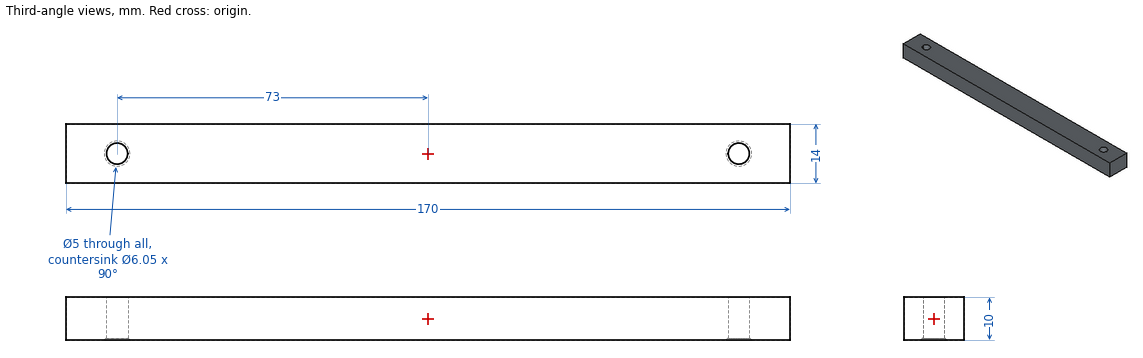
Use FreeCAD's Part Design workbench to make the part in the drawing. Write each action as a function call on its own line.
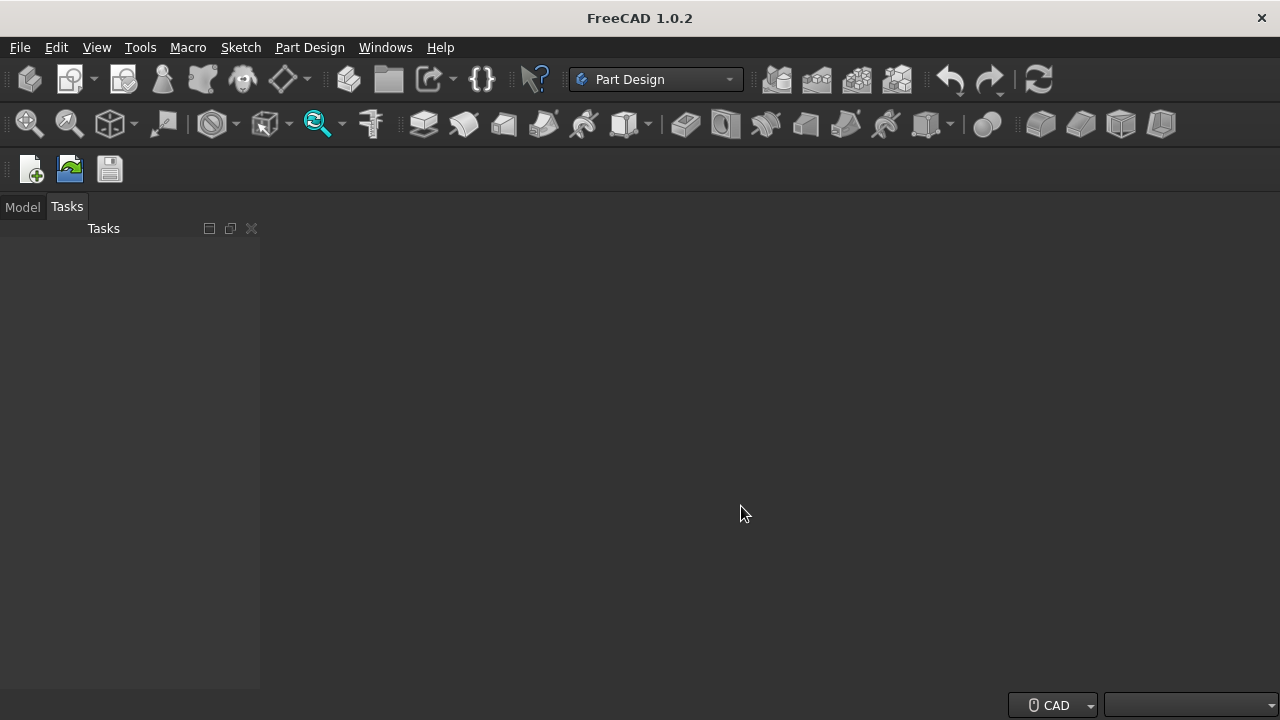
click(30, 170)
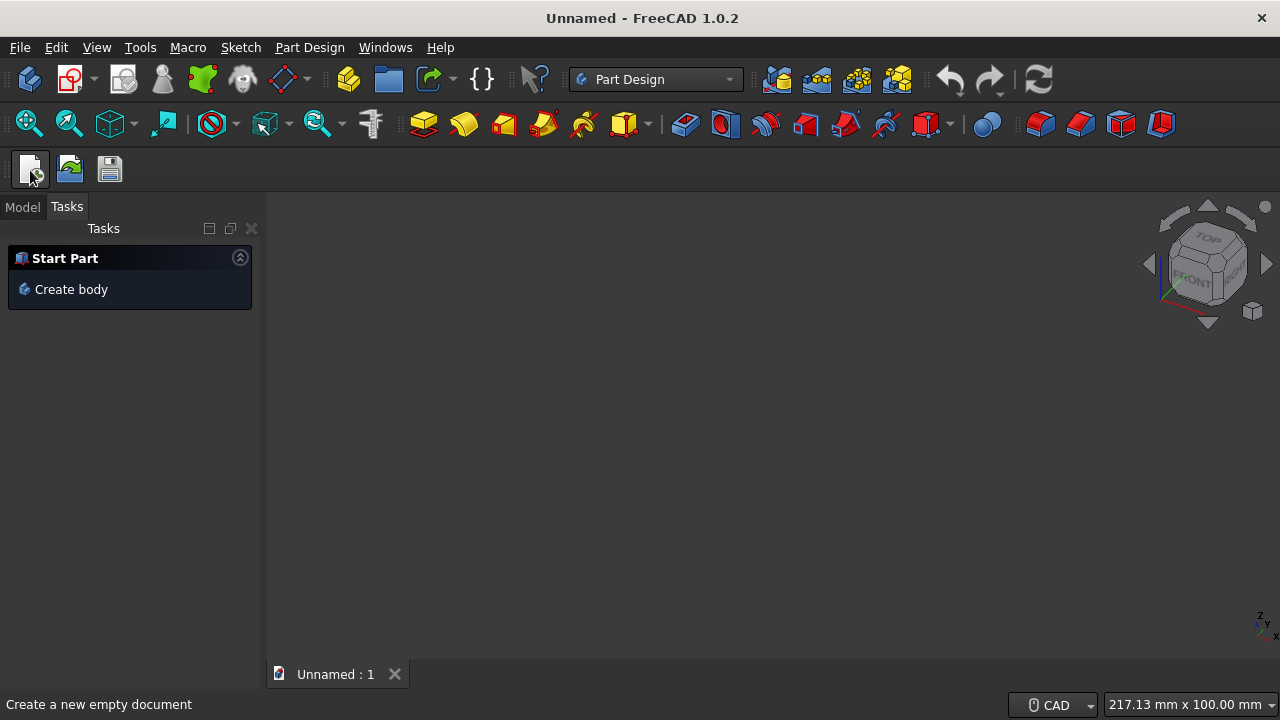
click(70, 80)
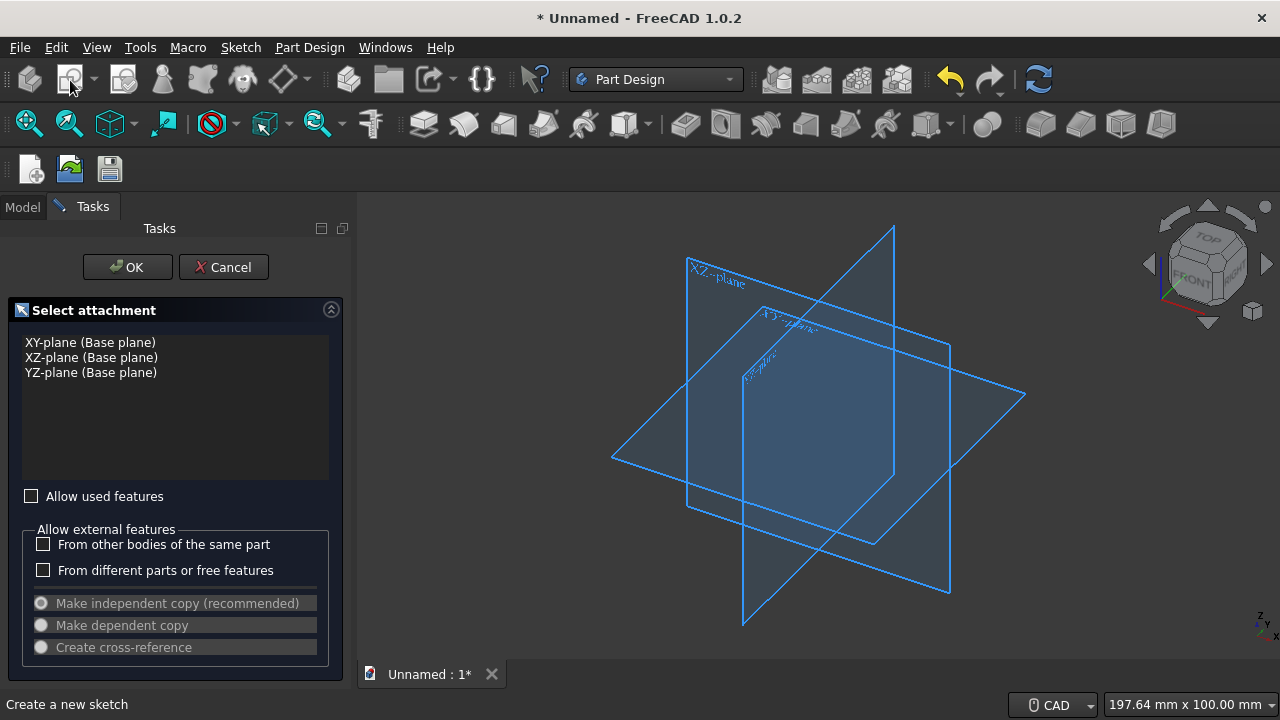
click(82, 342)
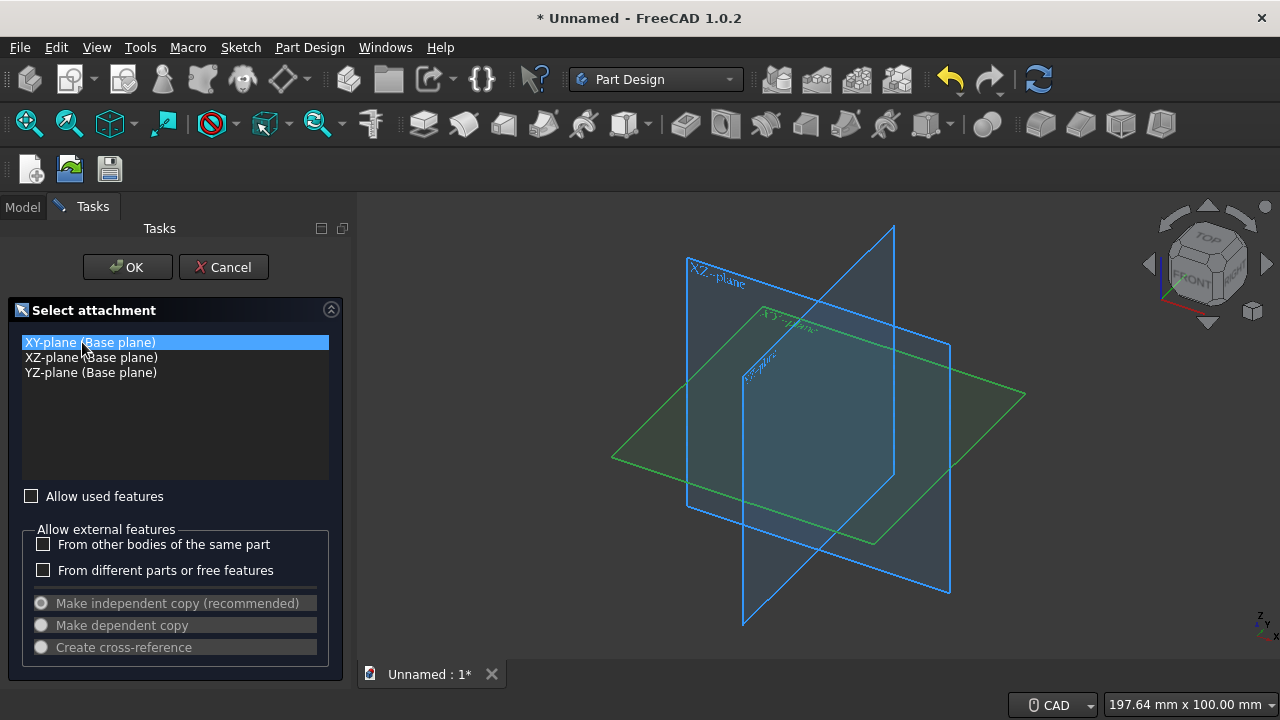
click(128, 267)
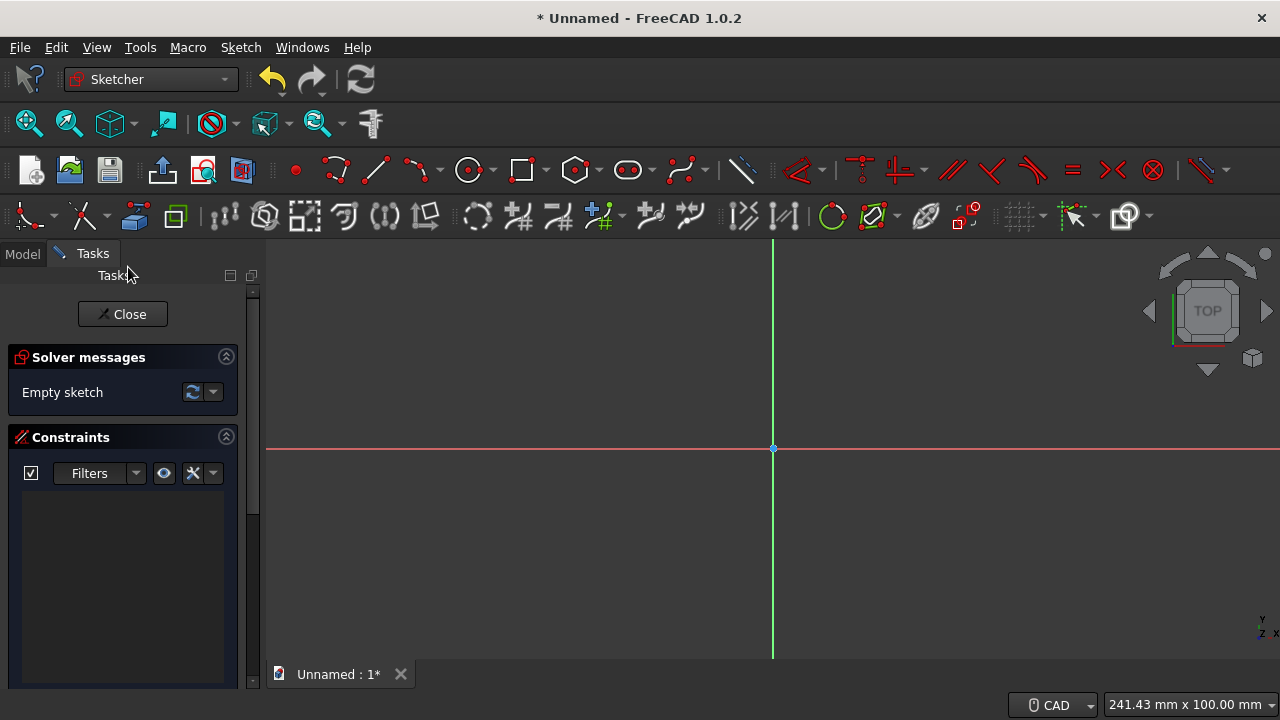
scroll(395, 449, down, 1)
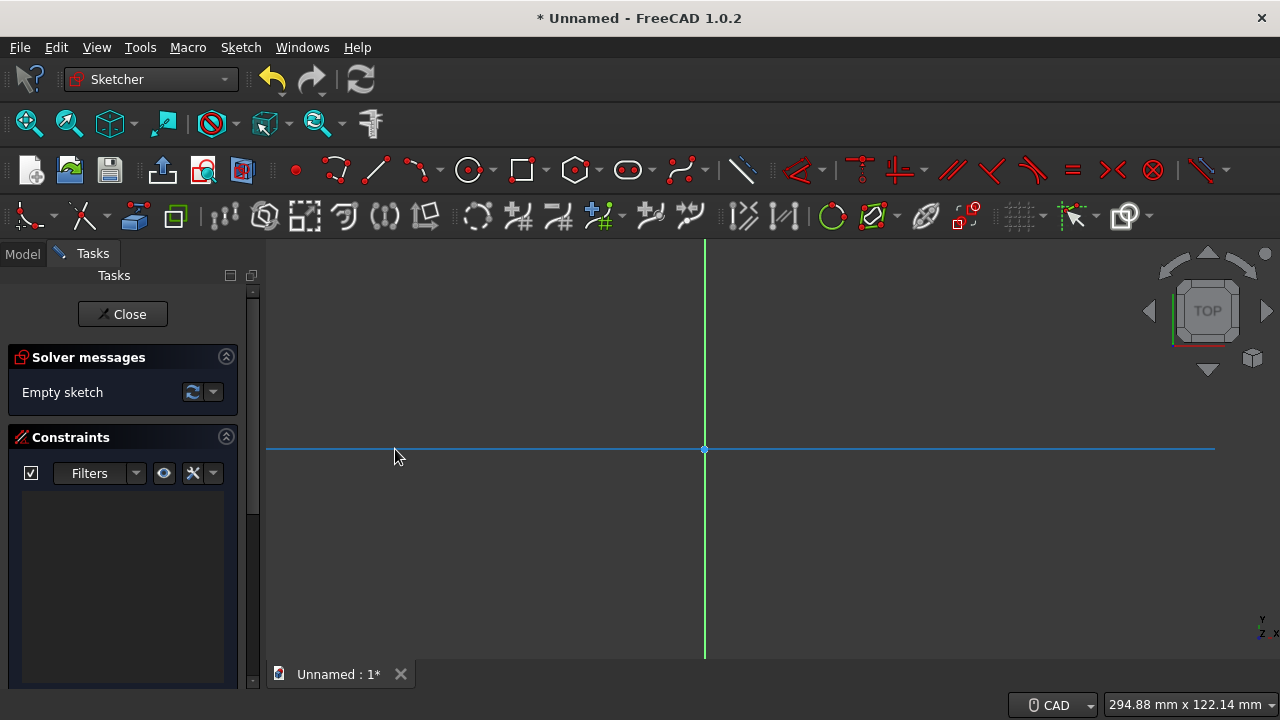
click(548, 170)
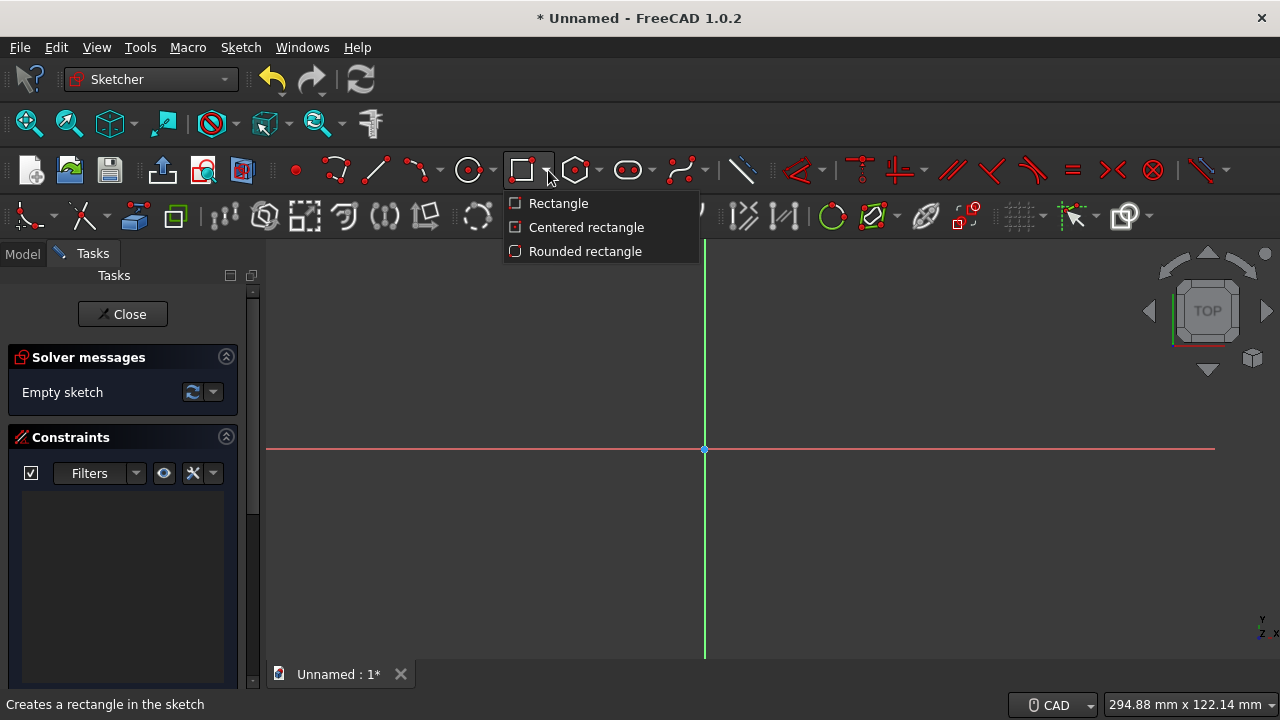
click(602, 227)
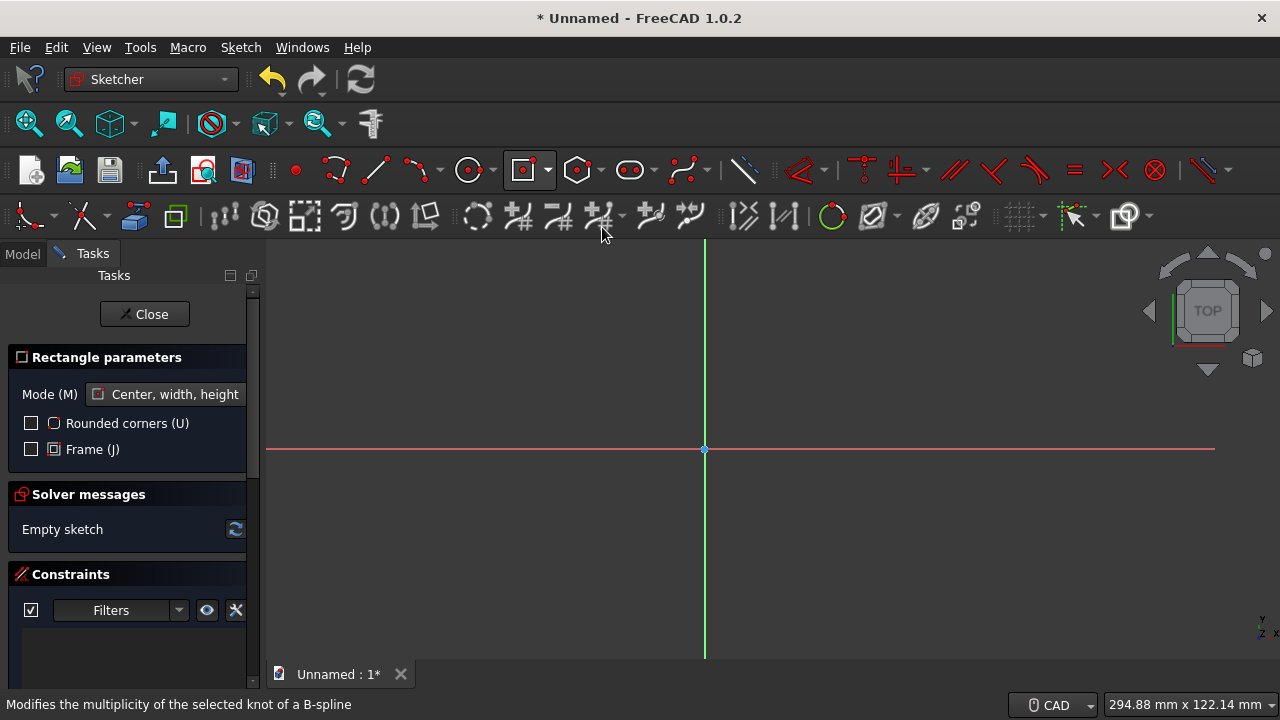
click(705, 449)
click(997, 425)
key(Escape)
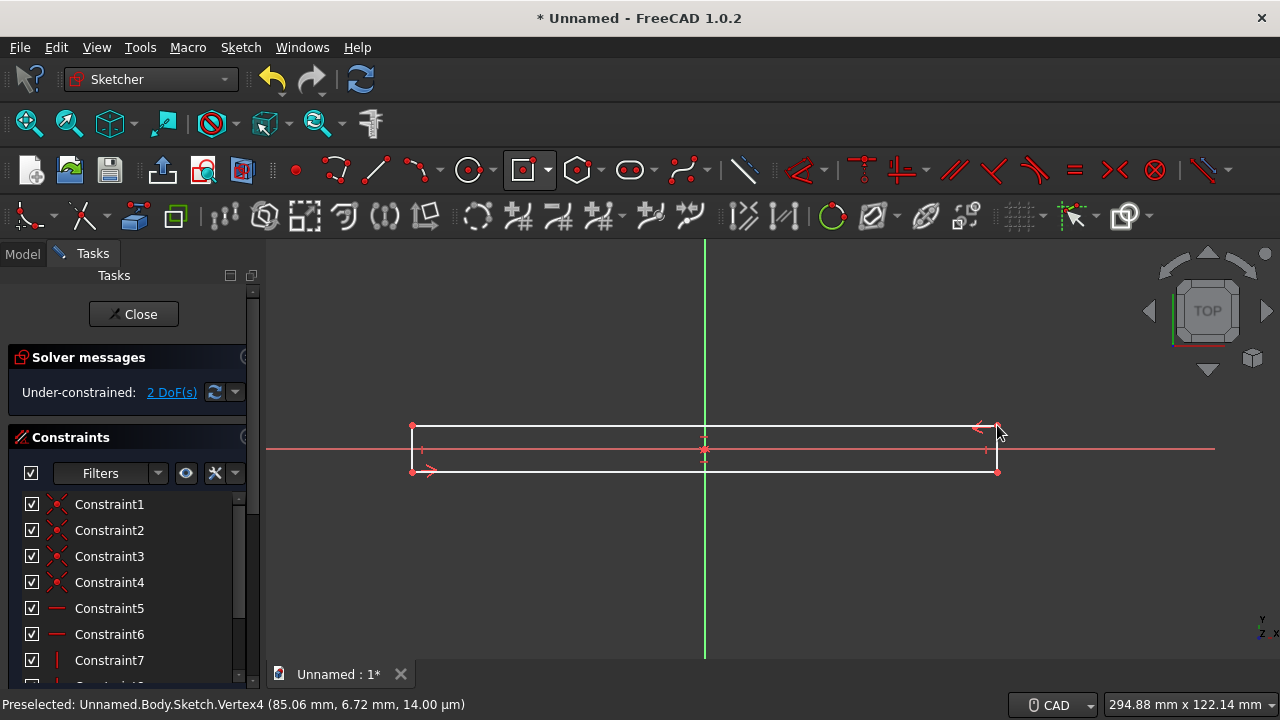
click(800, 170)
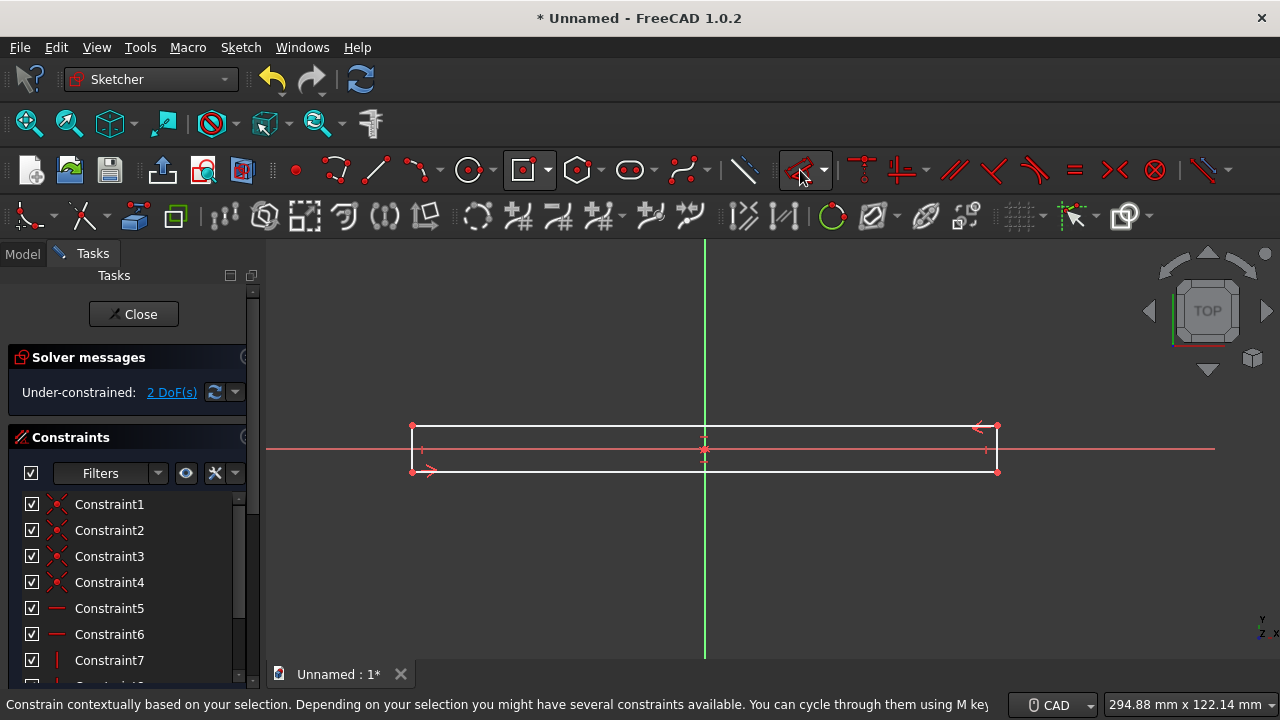
scroll(997, 458, up, 3)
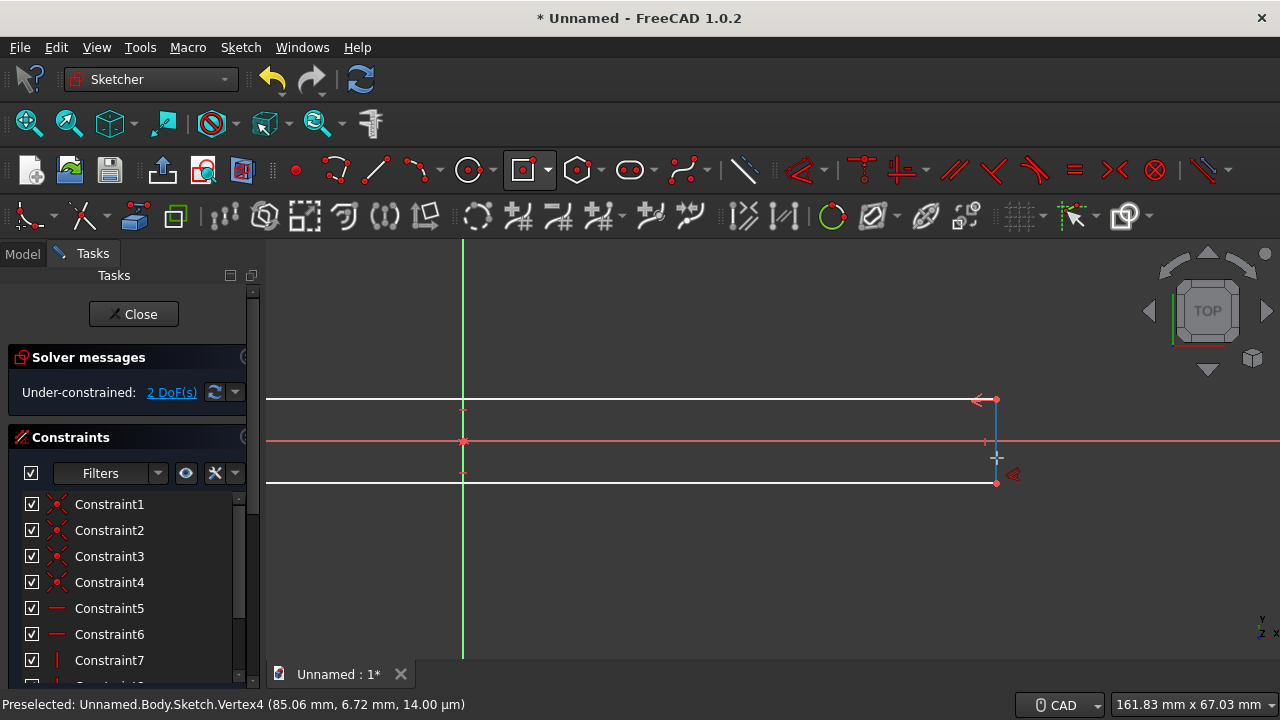
click(996, 458)
click(1030, 422)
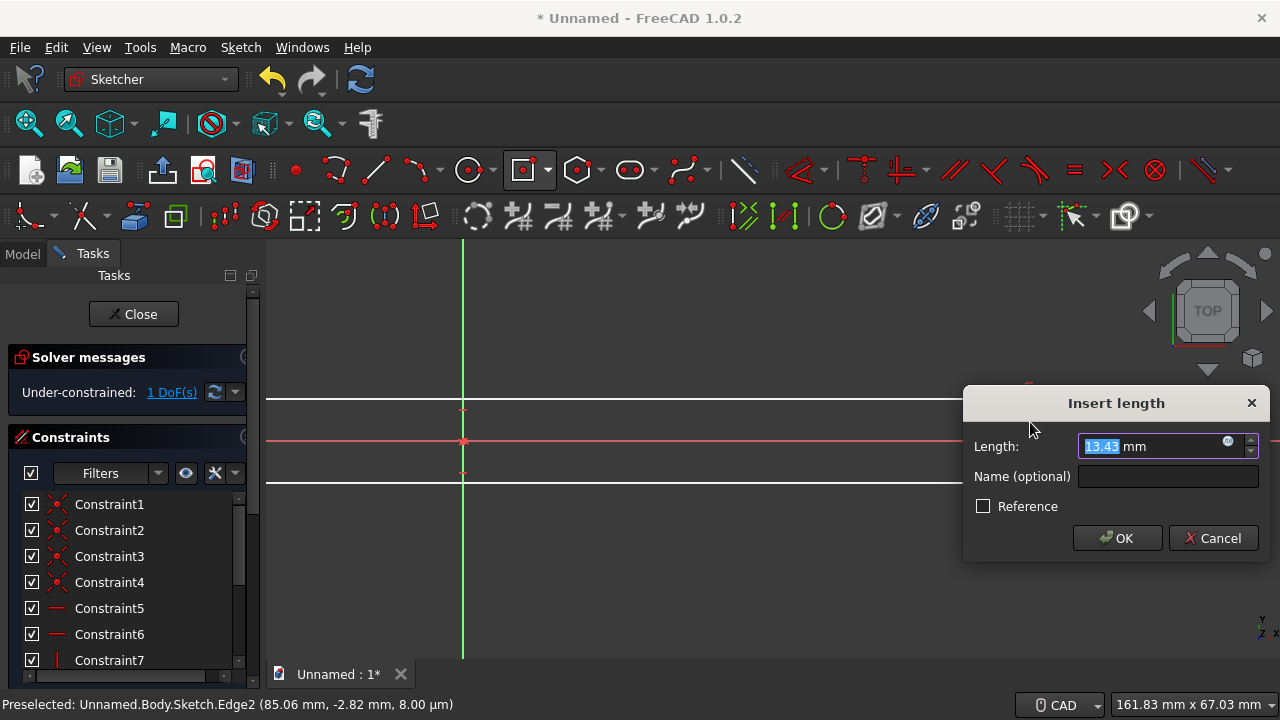
text(14)
key(Return)